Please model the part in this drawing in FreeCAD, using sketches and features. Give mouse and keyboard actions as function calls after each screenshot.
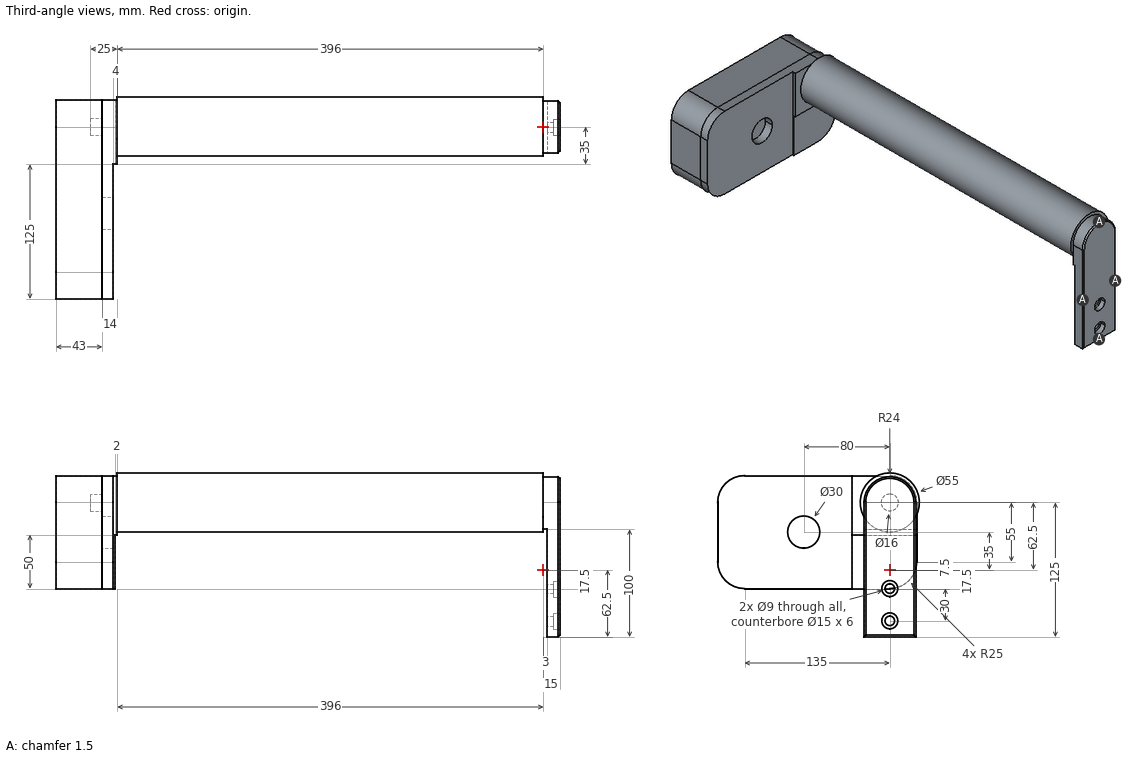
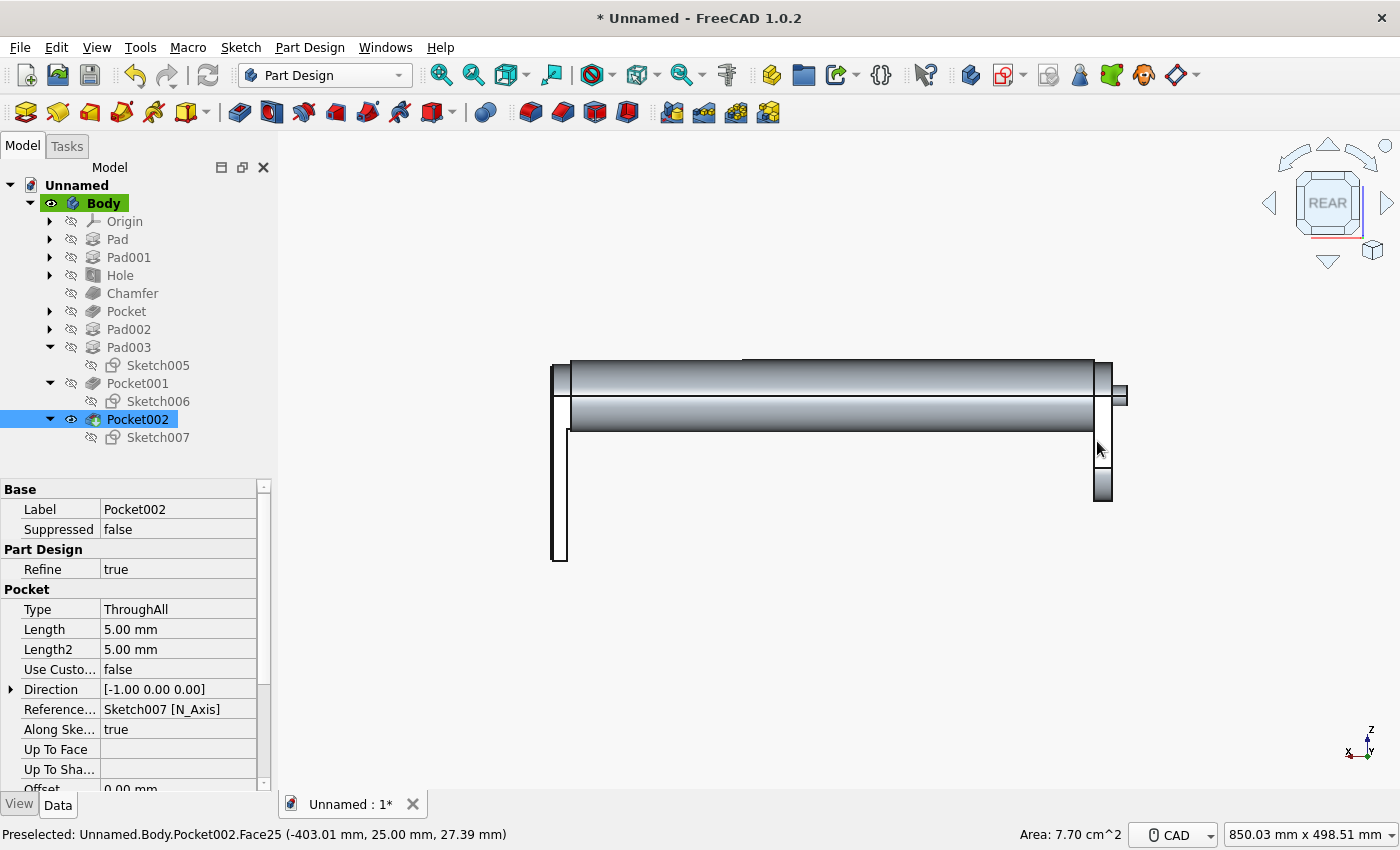
click(1004, 76)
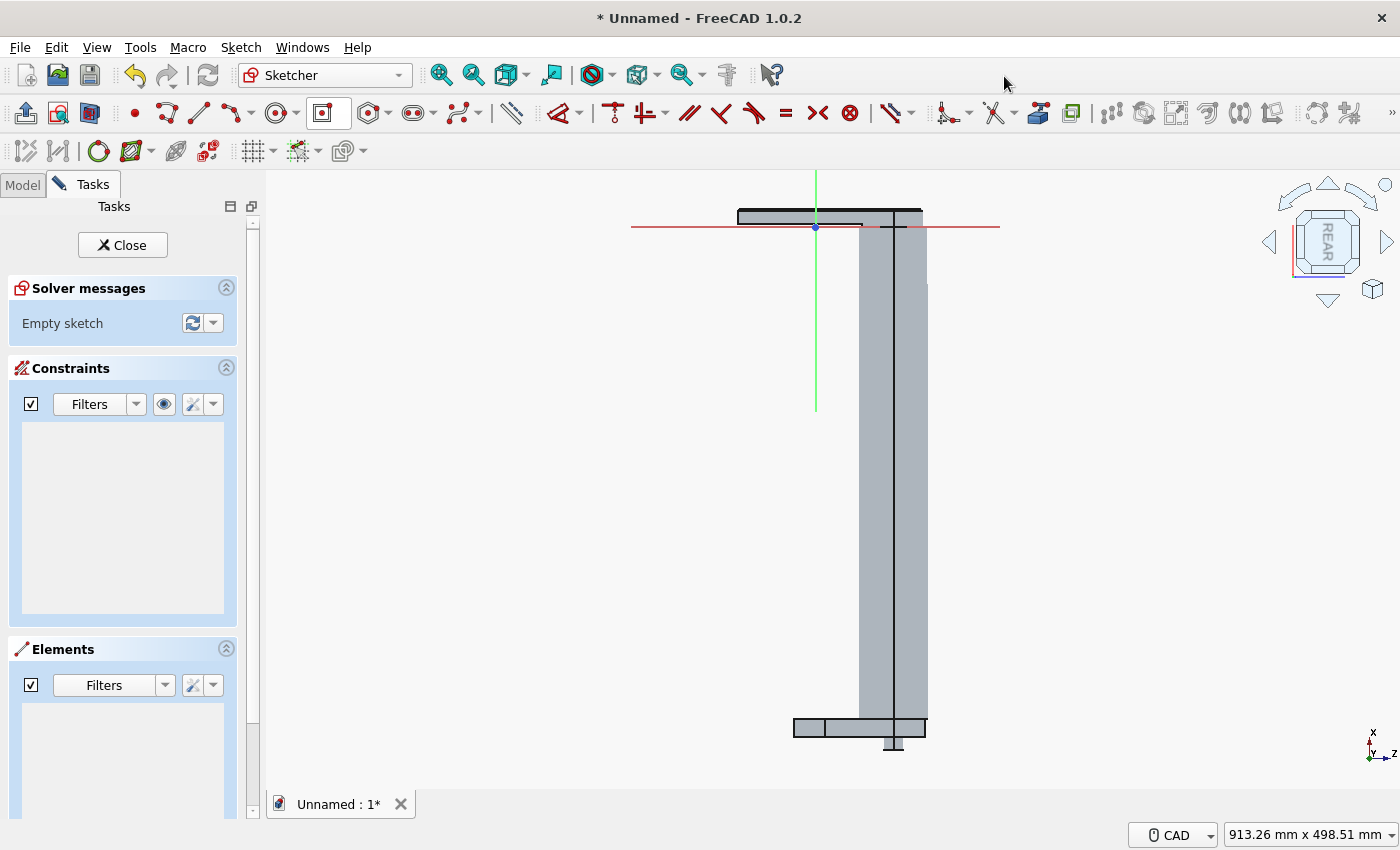
scroll(831, 744, up, 12)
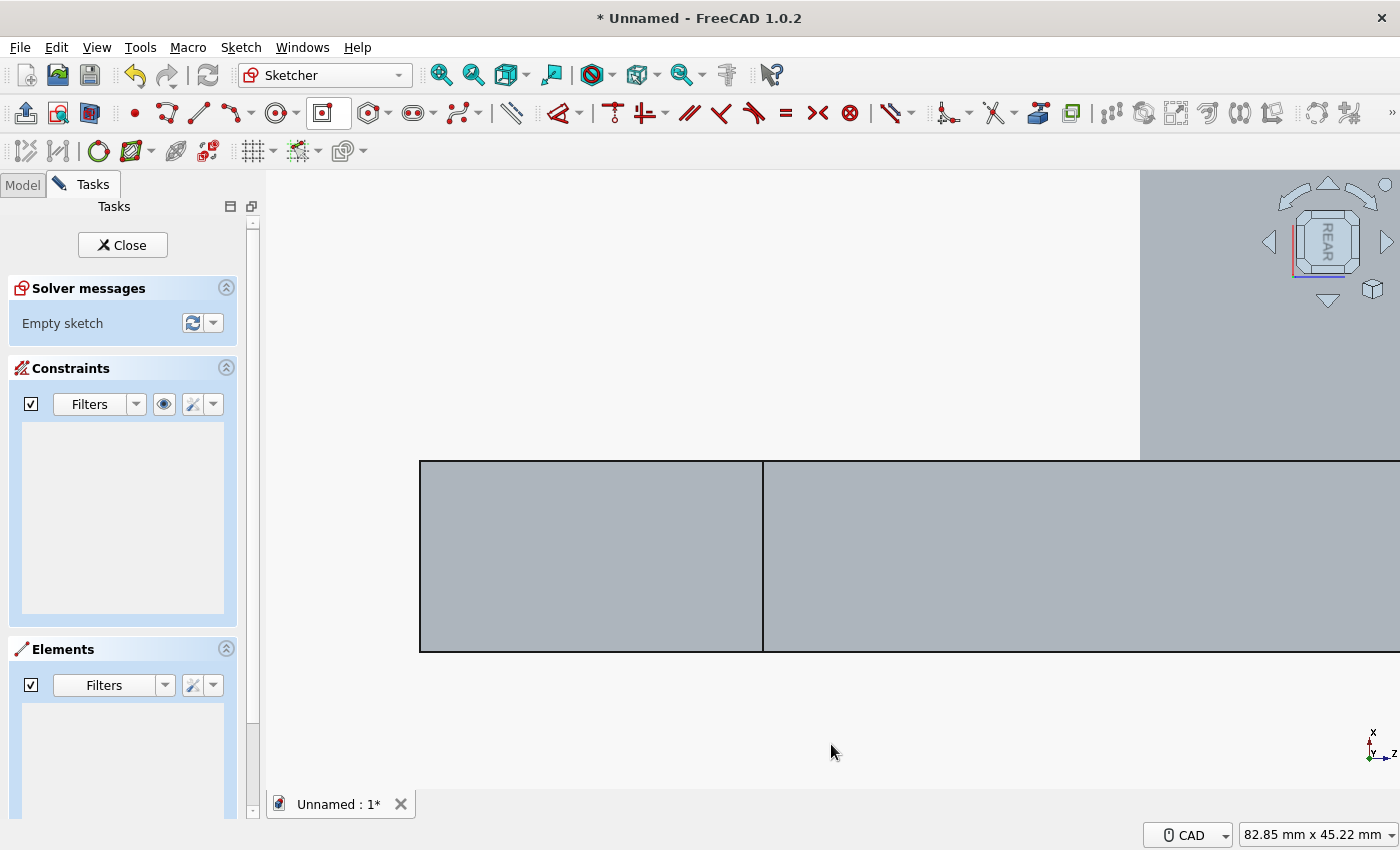
key(g)
key(r)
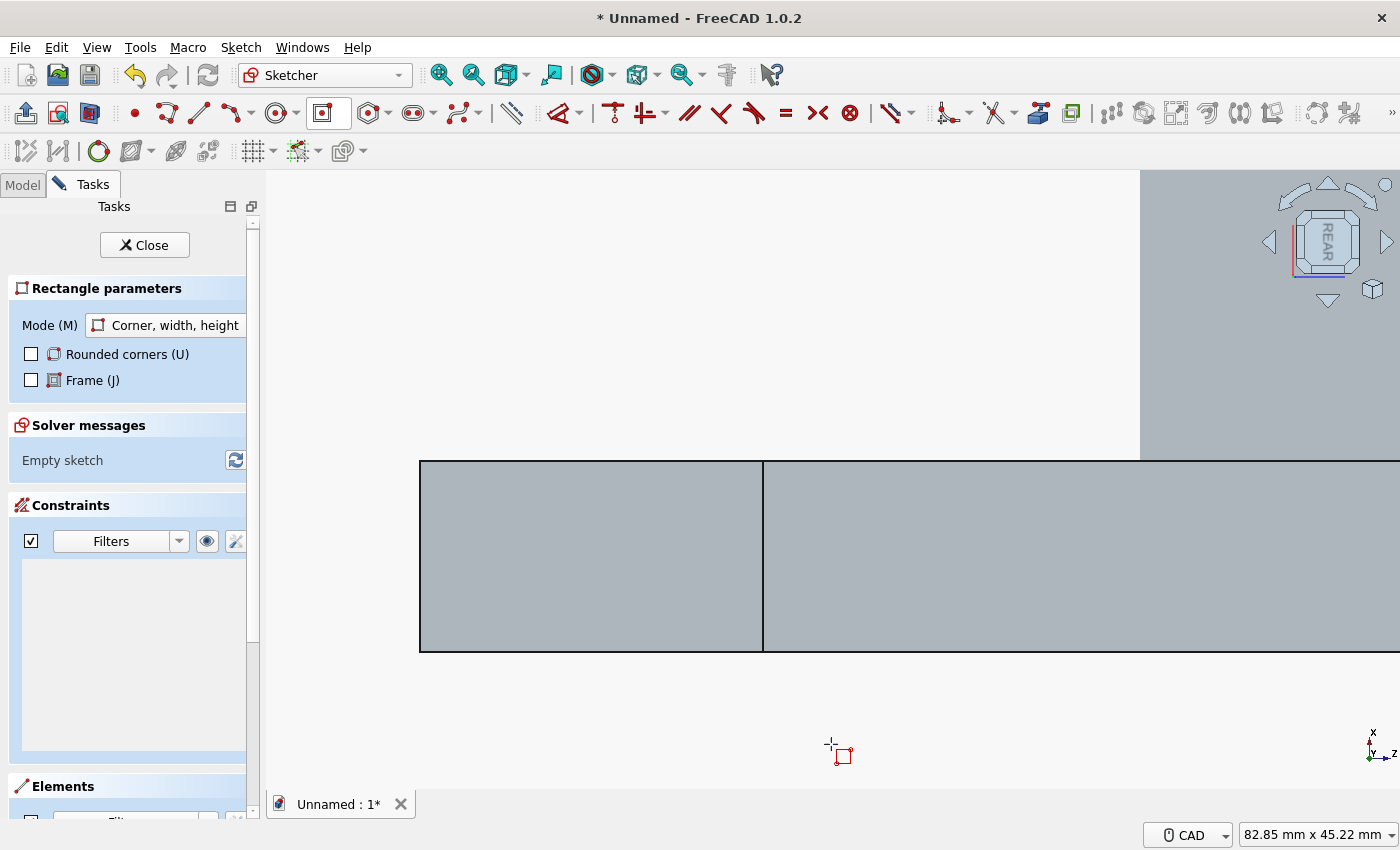
click(420, 461)
move(1105, 488)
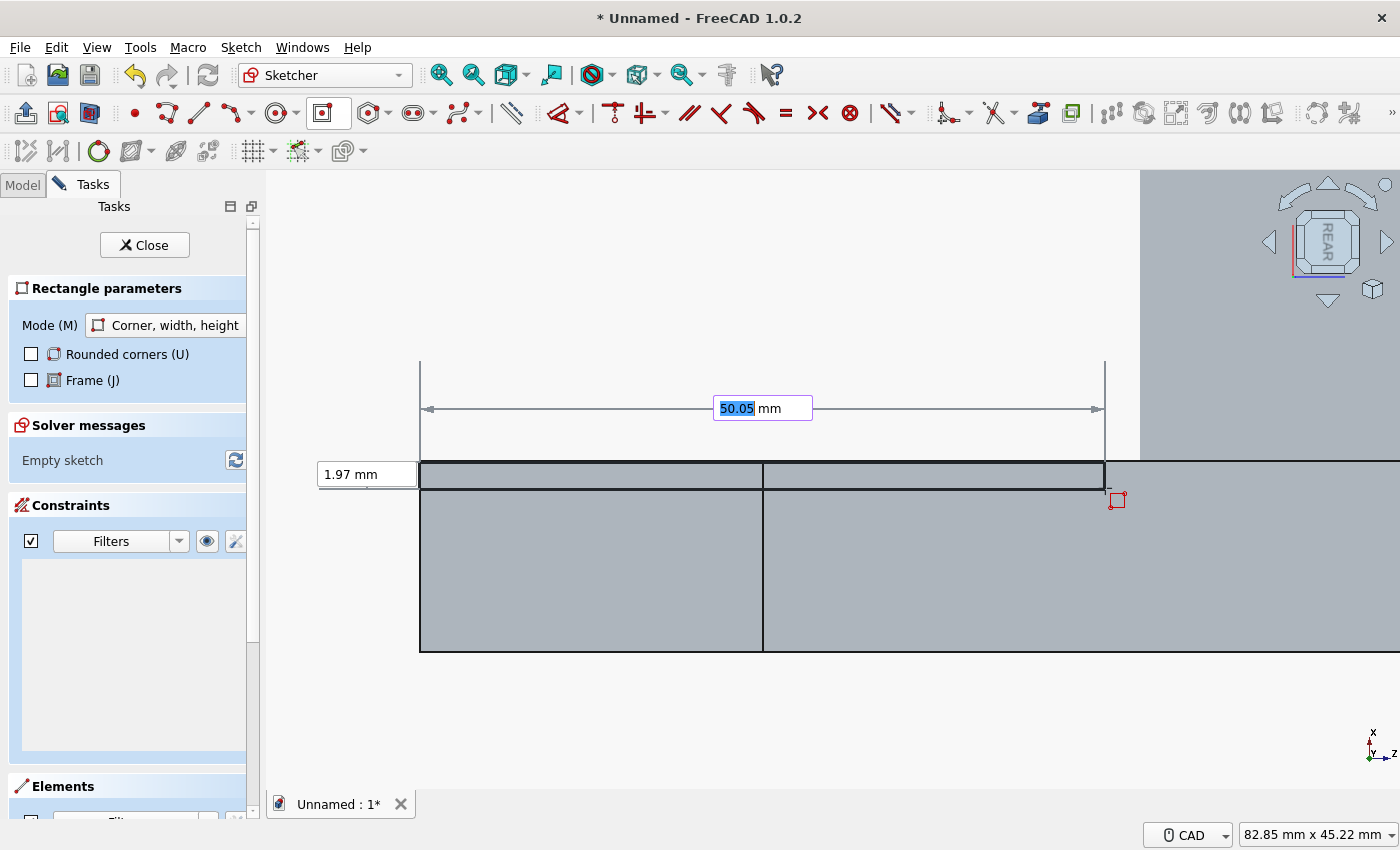
text(50)
key(Tab)
text(2)
key(Return)
key(Escape)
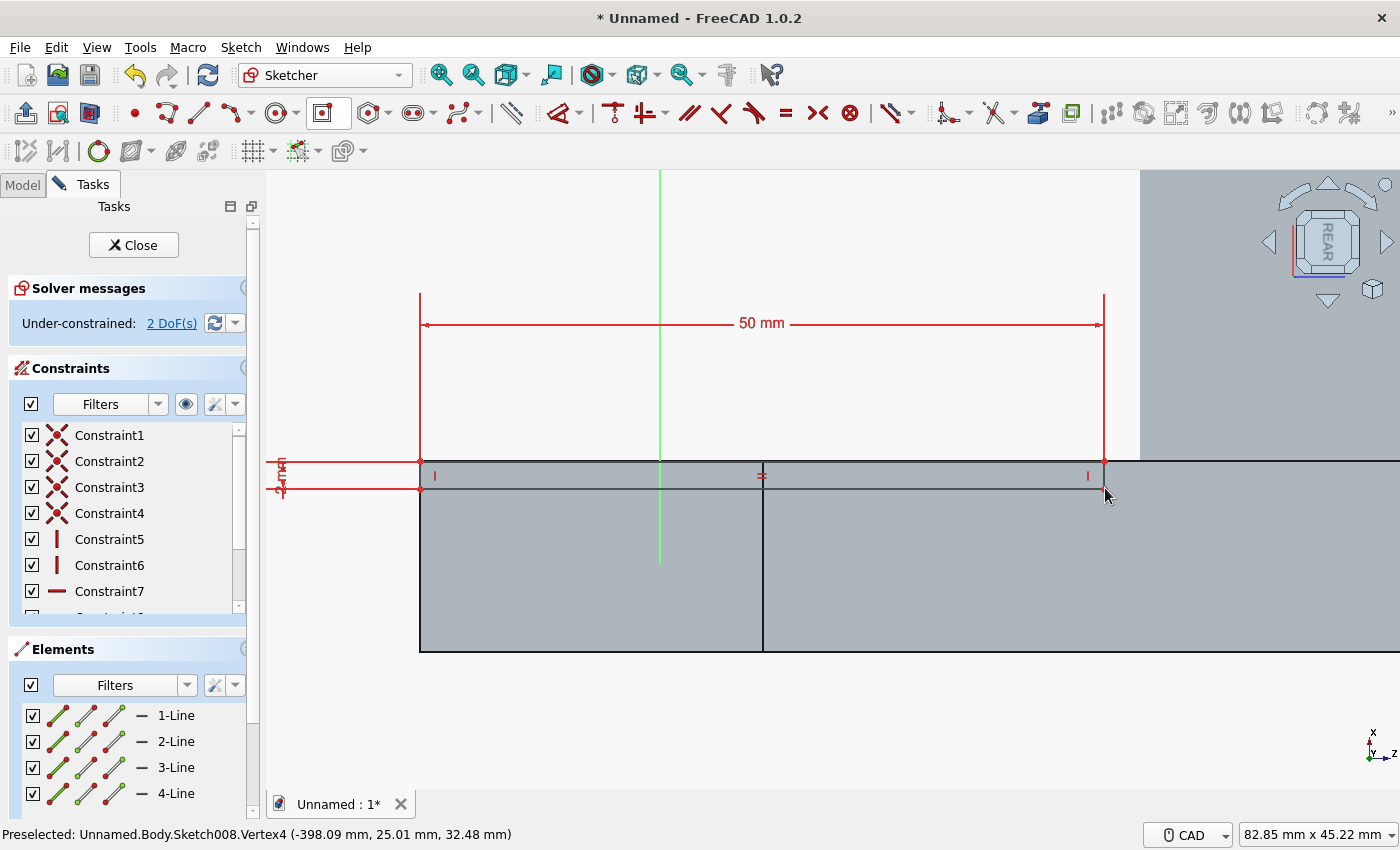
key(d)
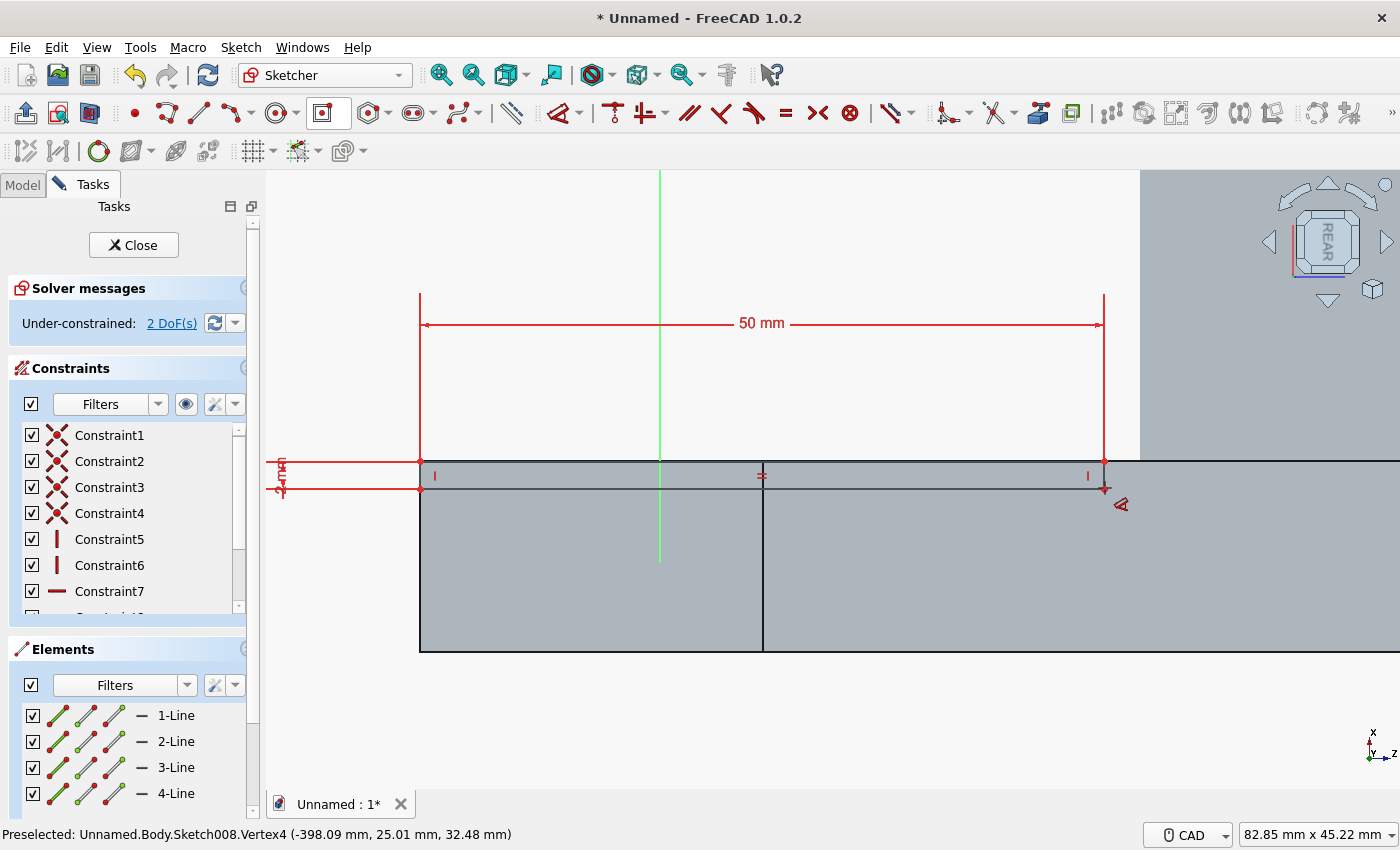
click(420, 462)
click(386, 330)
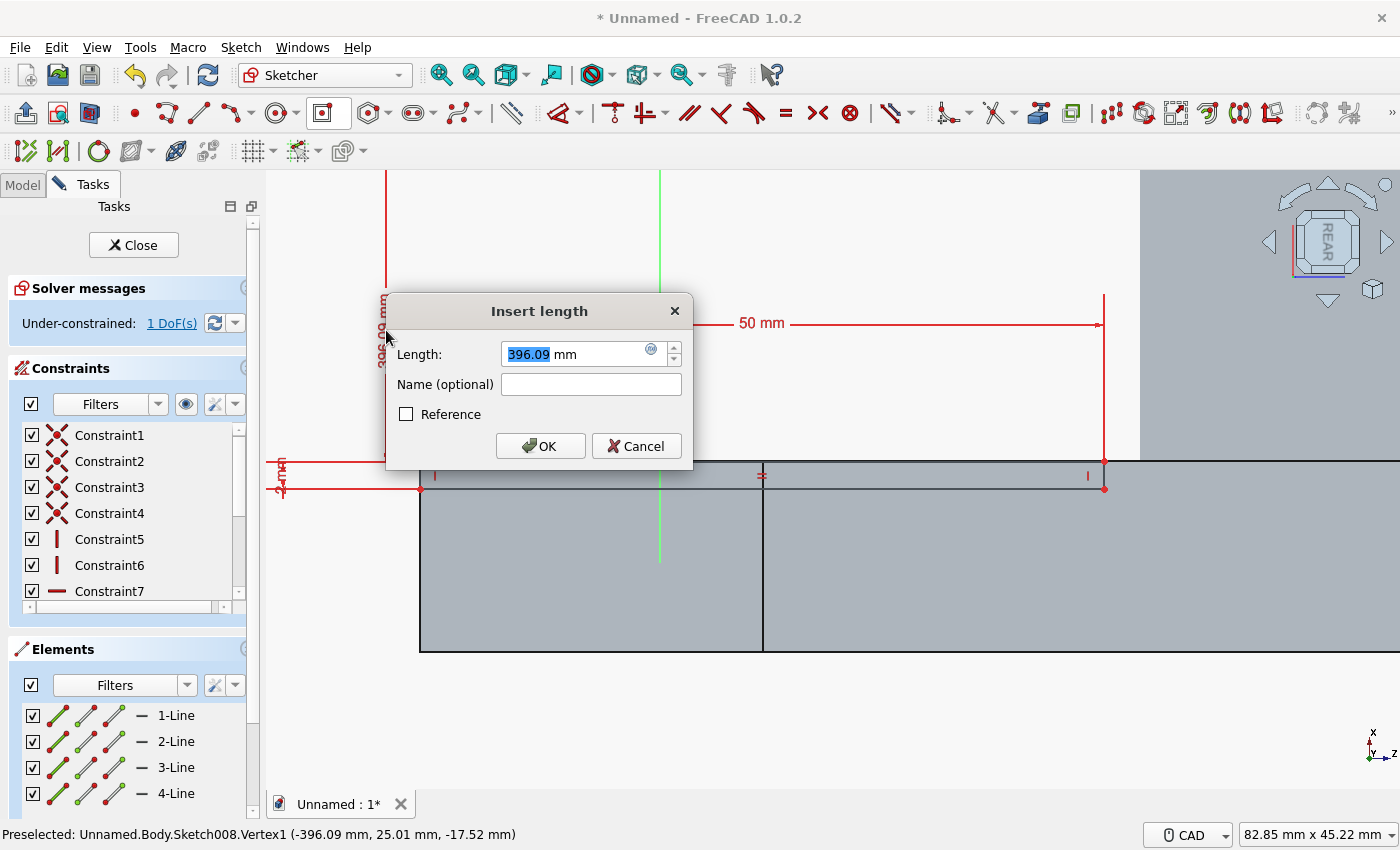
text(396)
key(Return)